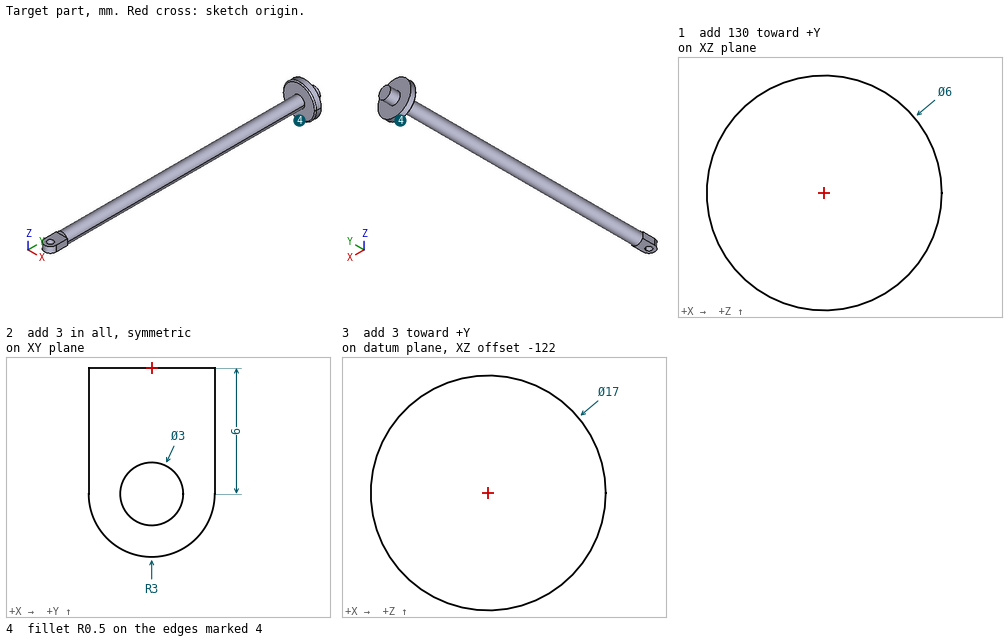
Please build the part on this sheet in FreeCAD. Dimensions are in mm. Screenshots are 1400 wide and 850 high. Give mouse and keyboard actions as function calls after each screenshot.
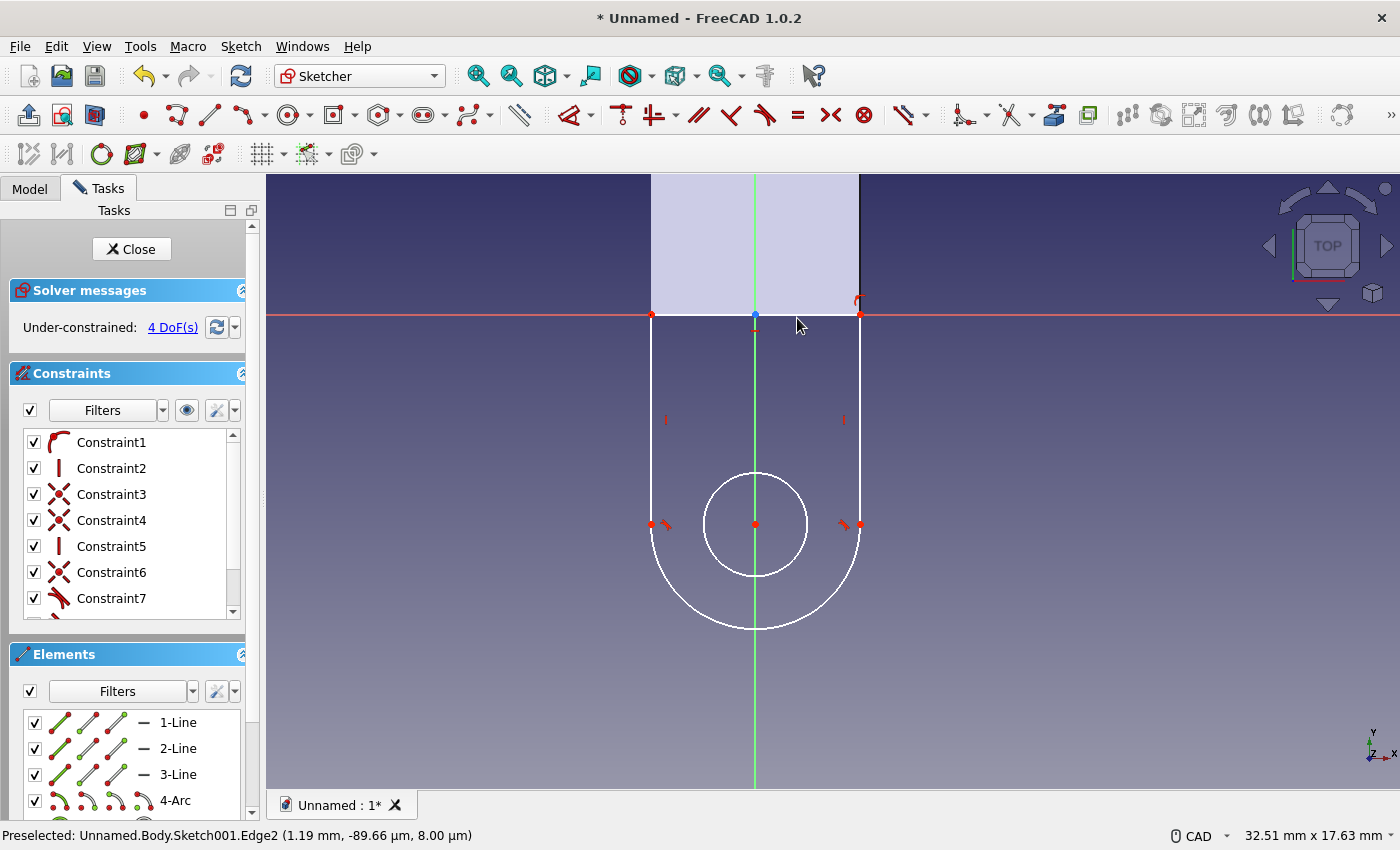
click(756, 525)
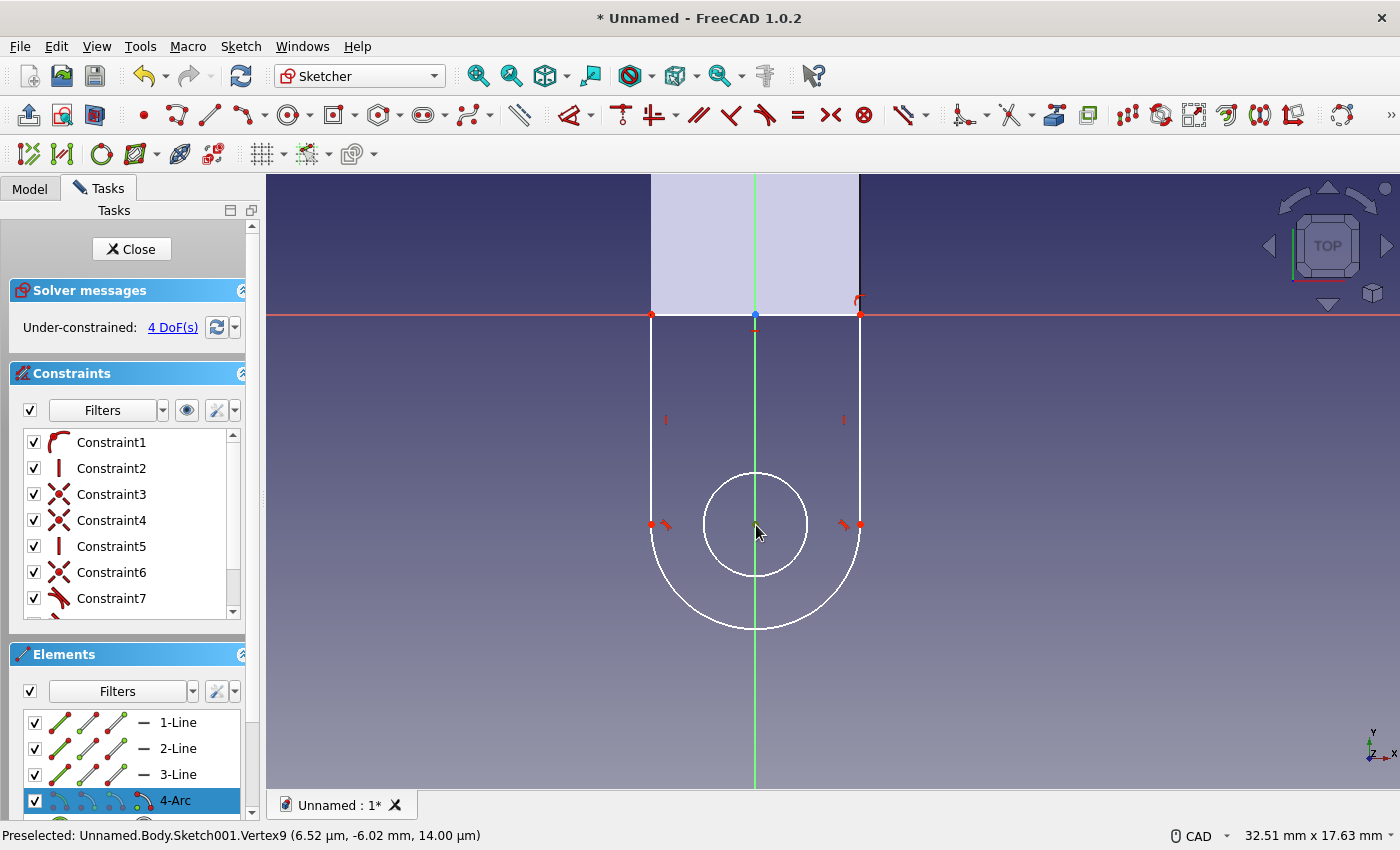
click(755, 721)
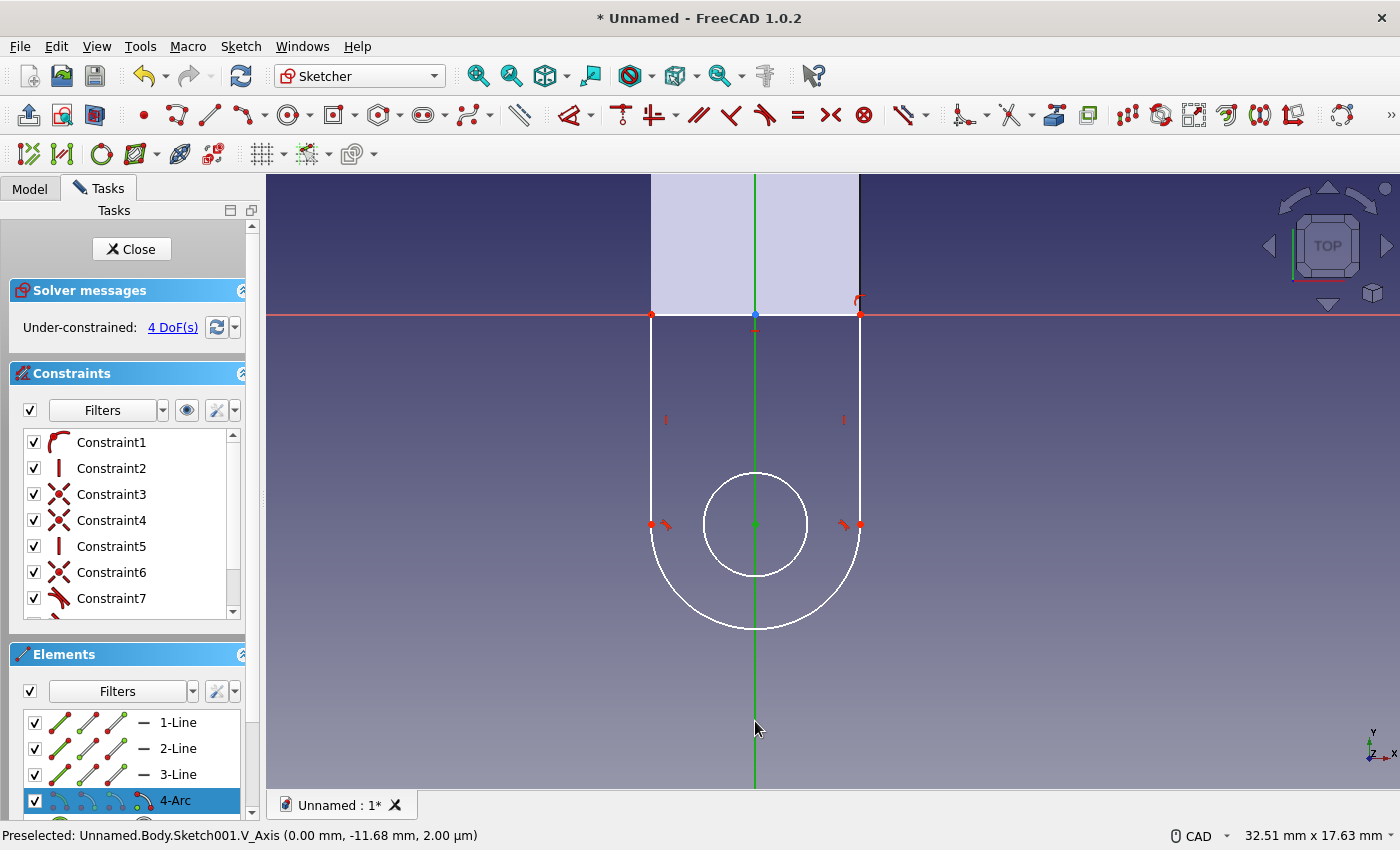
click(621, 116)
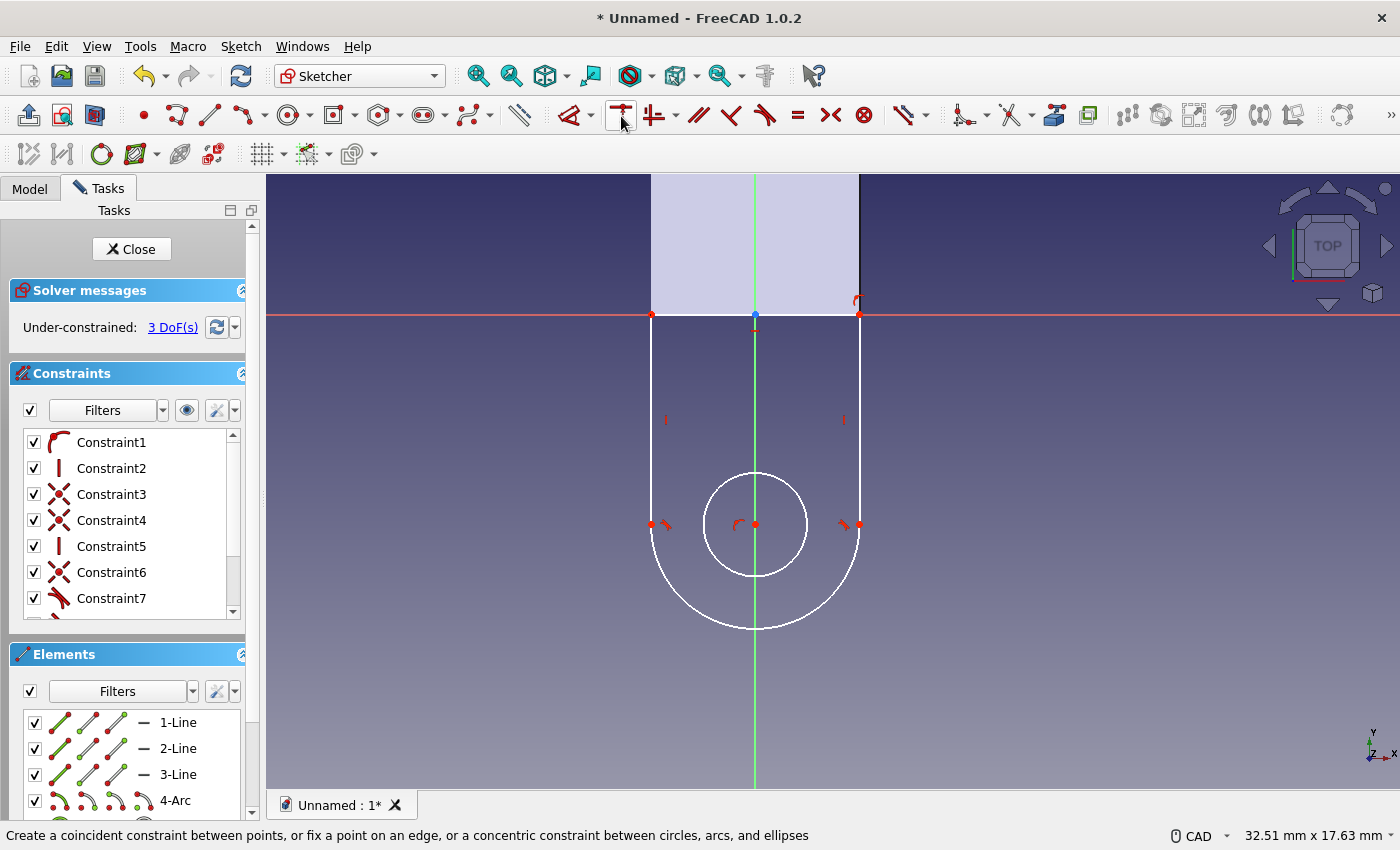
key(d)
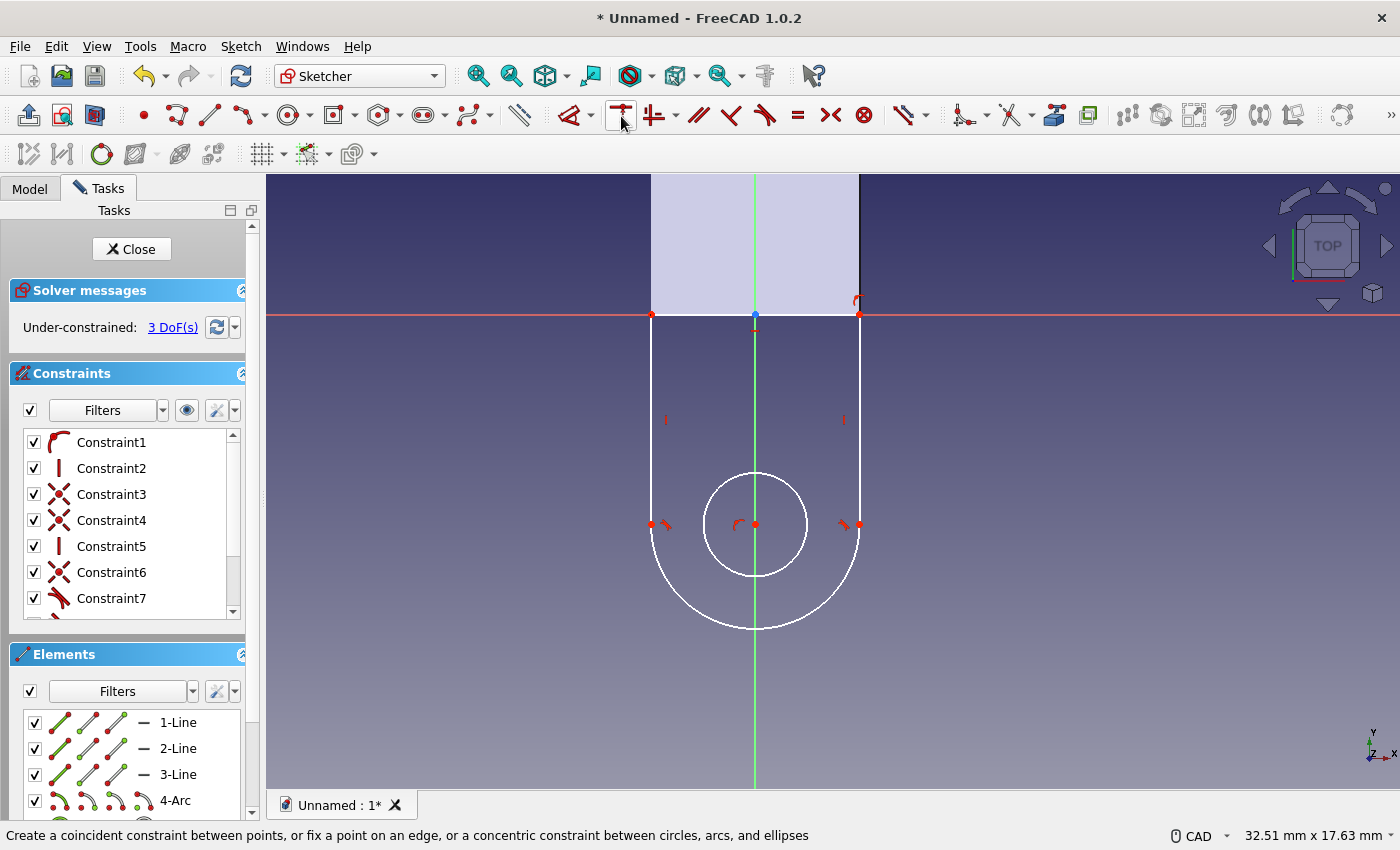
click(694, 609)
click(675, 635)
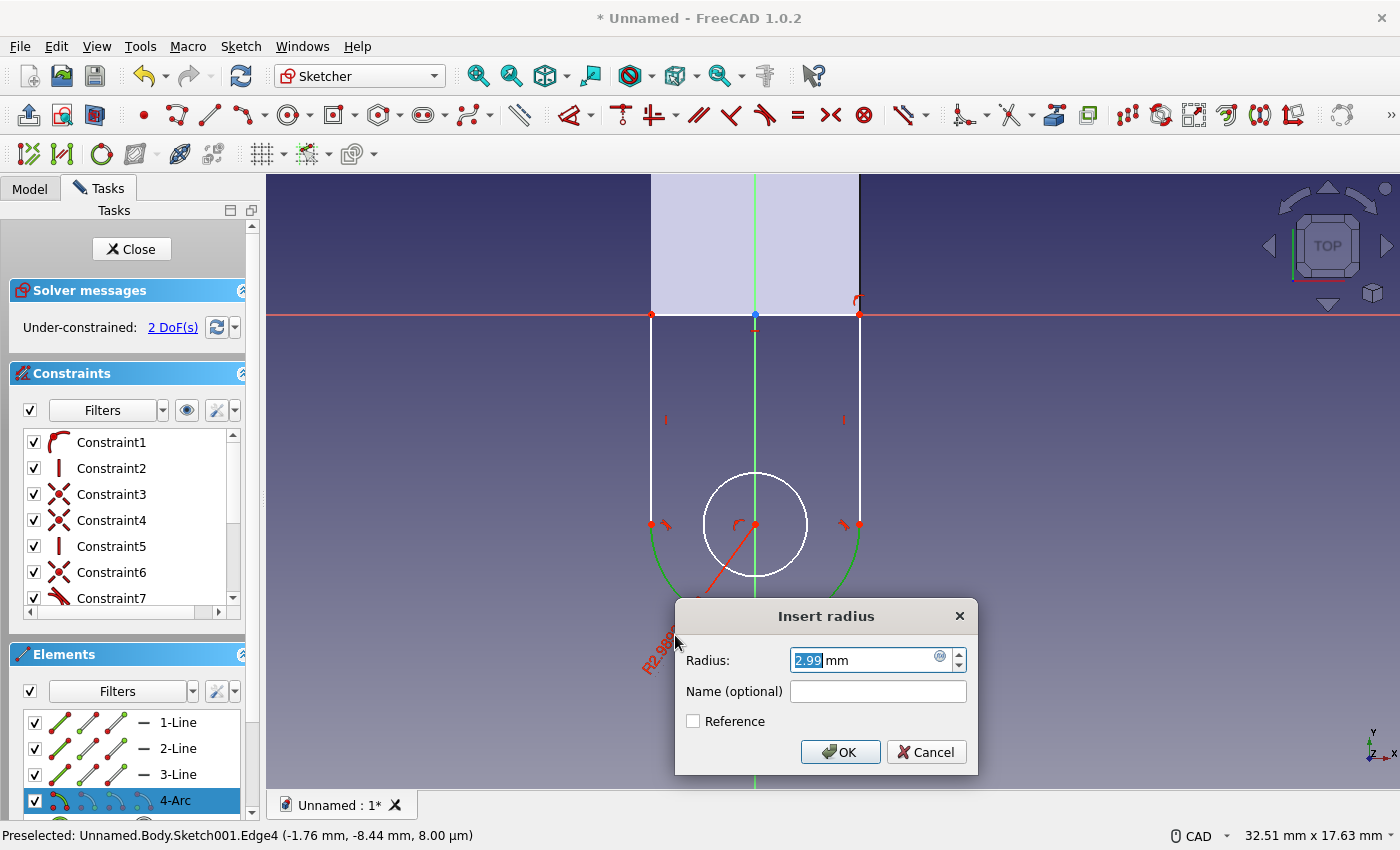
text(3)
key(Return)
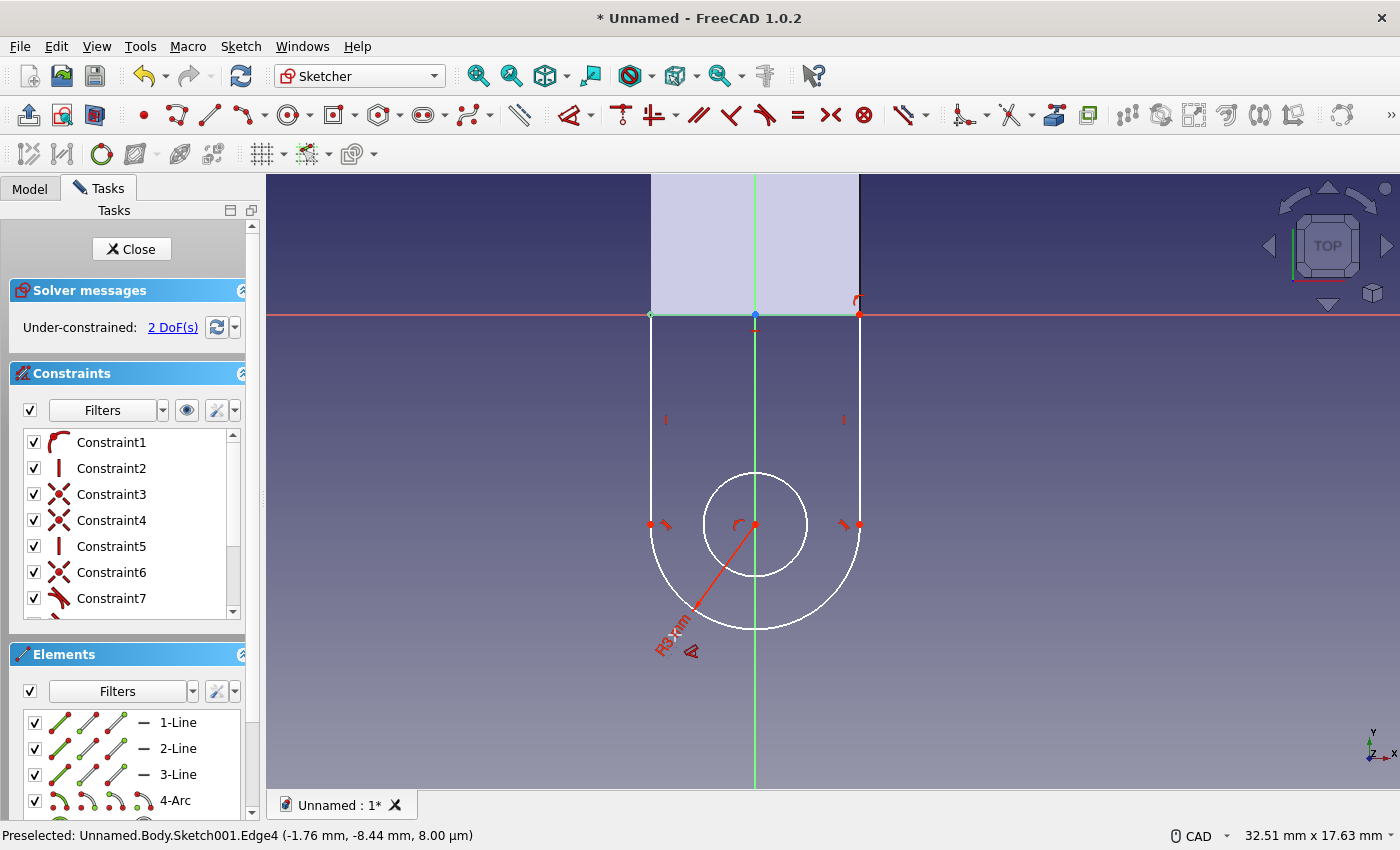
click(792, 488)
click(815, 465)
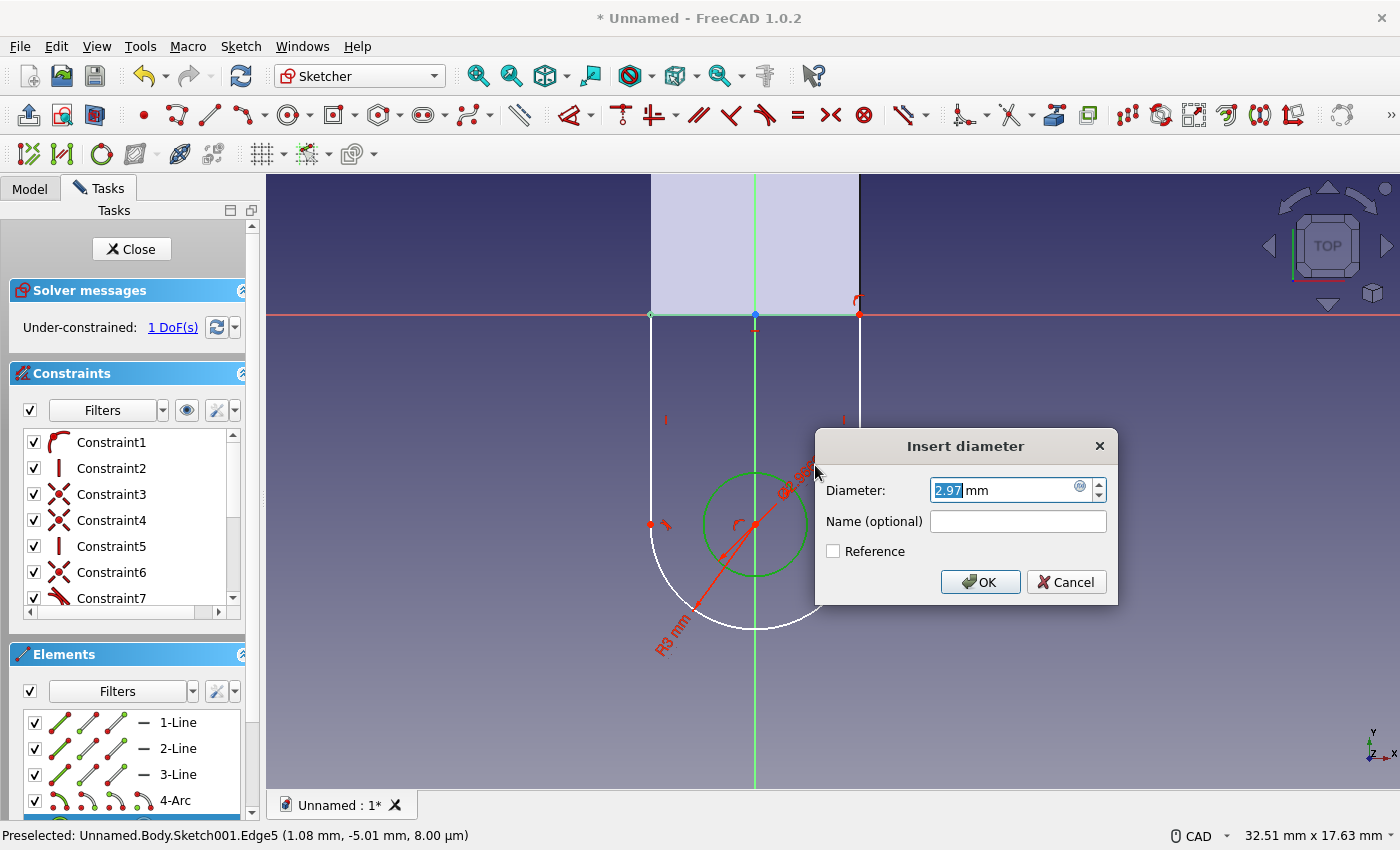
text(3)
key(Return)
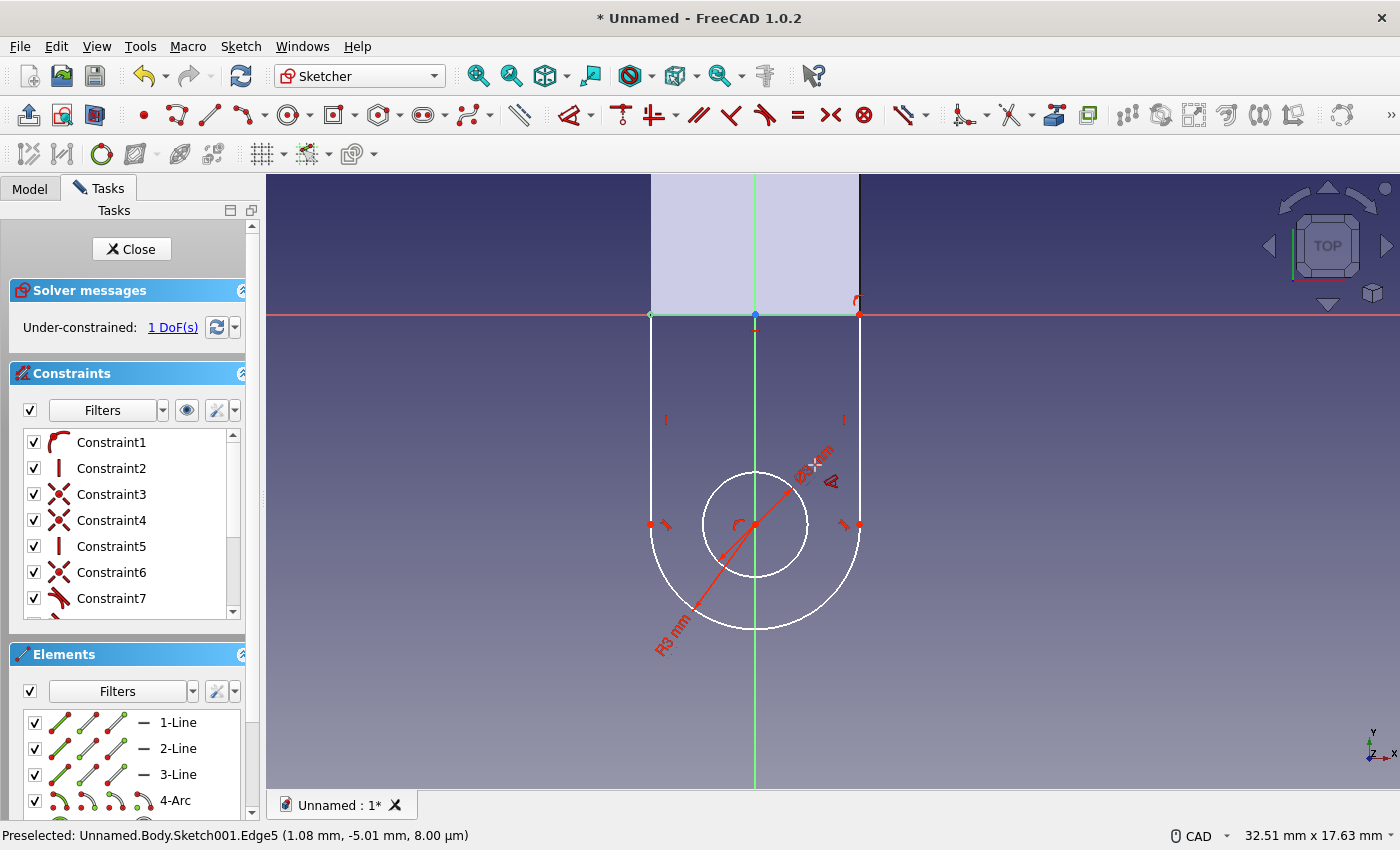
click(860, 462)
click(894, 420)